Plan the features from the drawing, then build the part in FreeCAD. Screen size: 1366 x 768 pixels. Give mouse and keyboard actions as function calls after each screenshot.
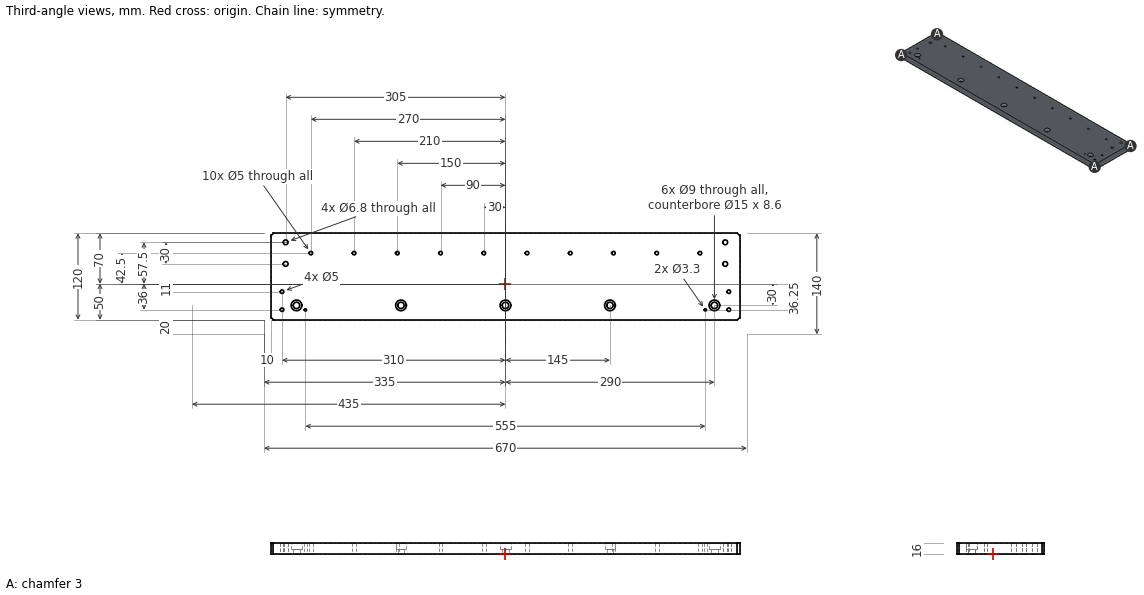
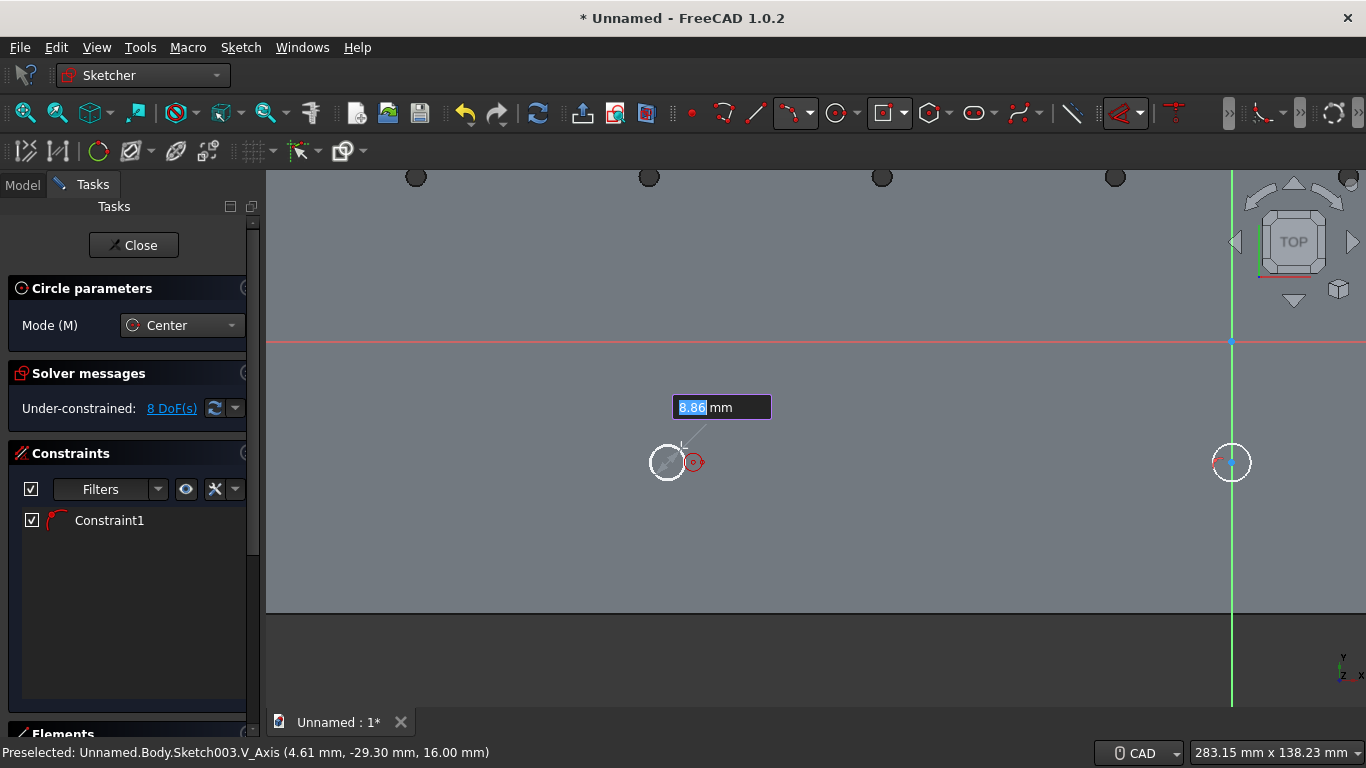
click(681, 446)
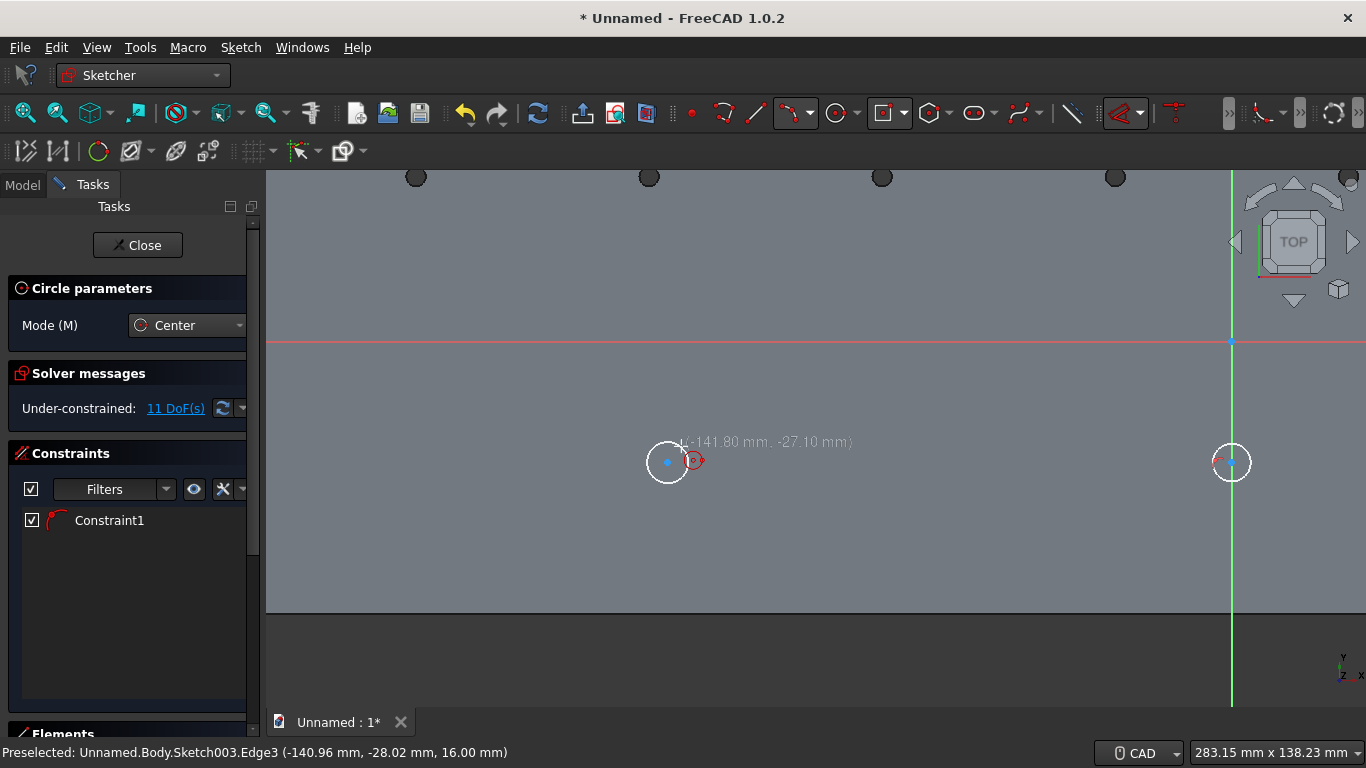
scroll(681, 448, down, 7)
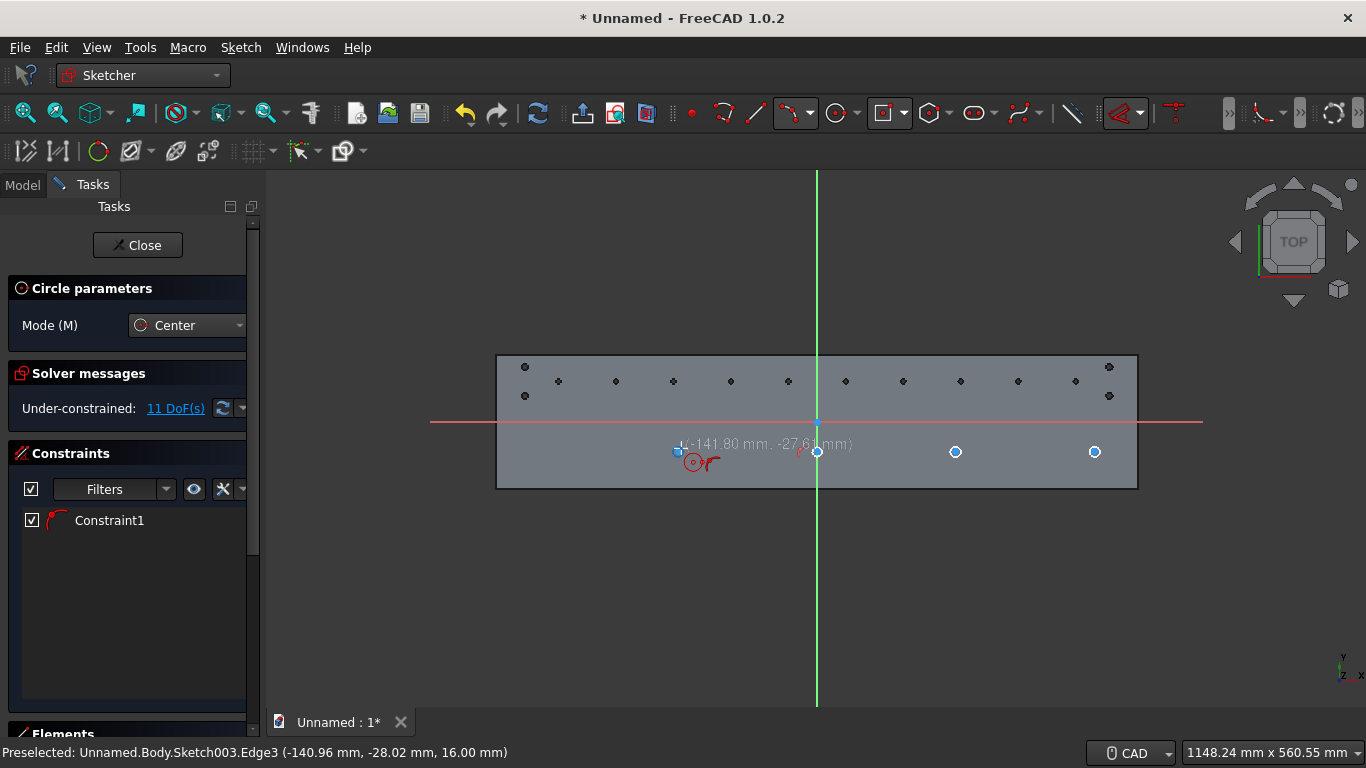
scroll(539, 451, up, 9)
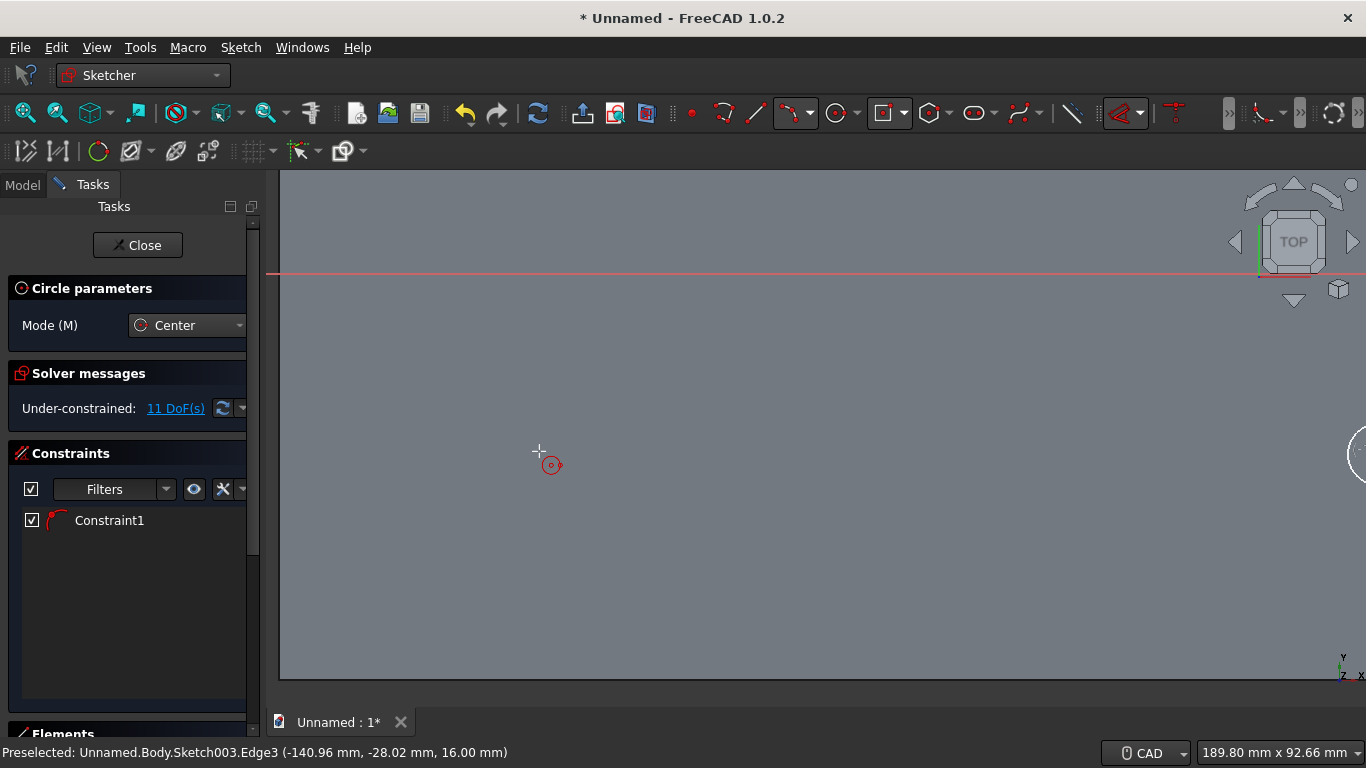
scroll(539, 451, down, 9)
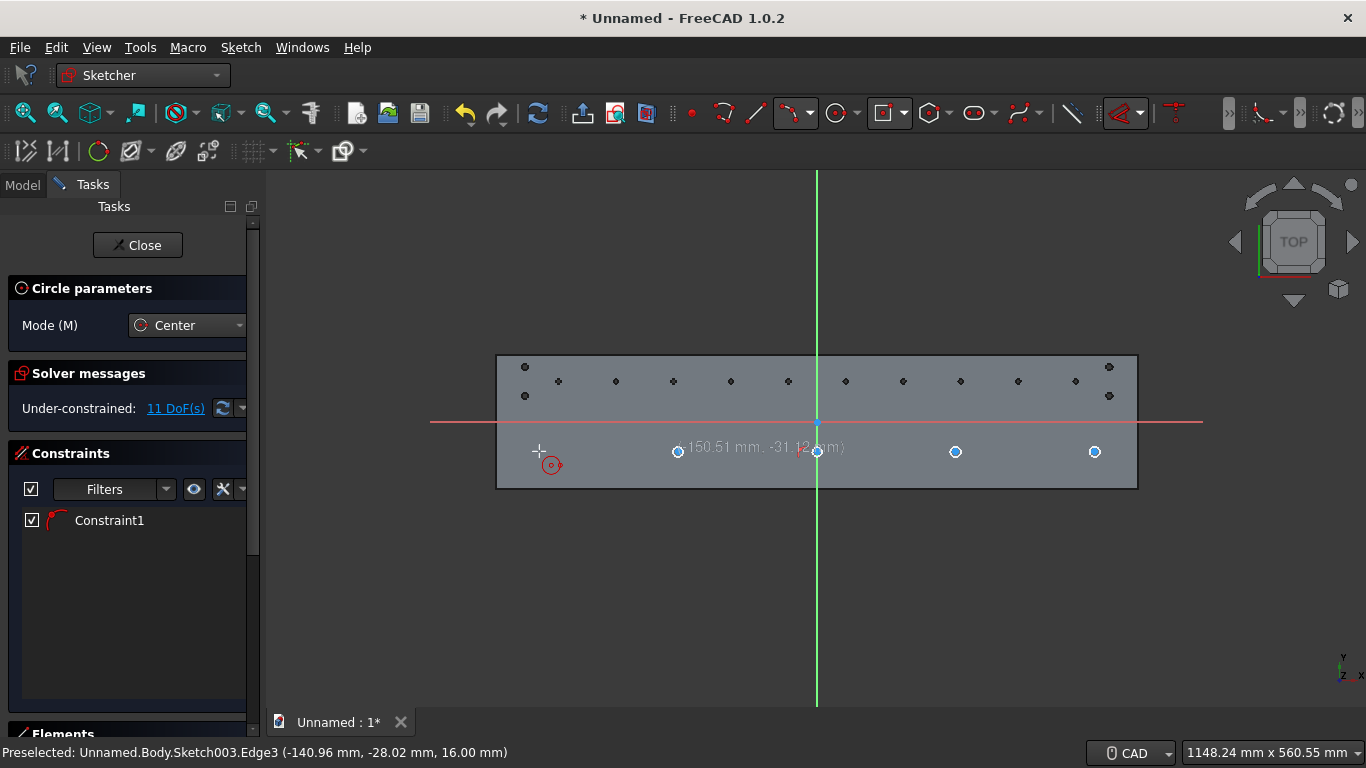
click(539, 451)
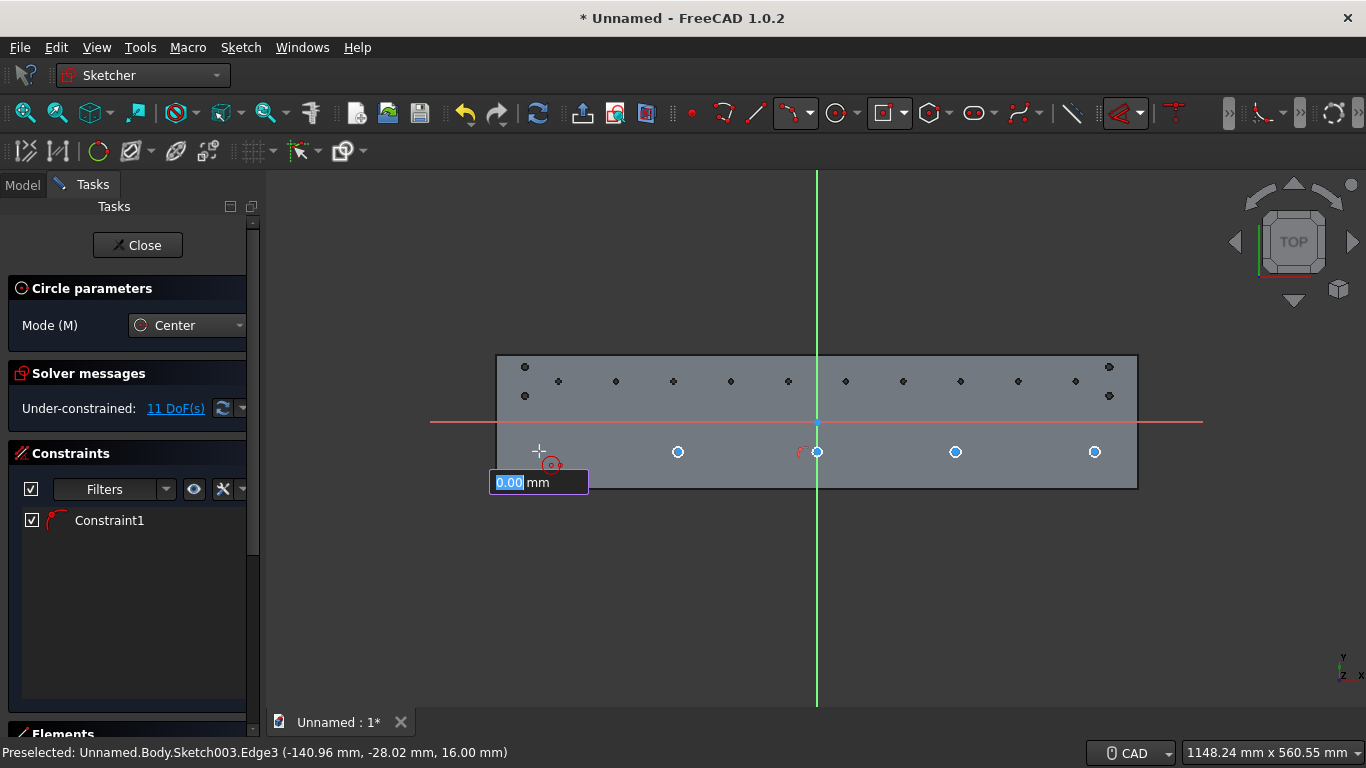
scroll(542, 448, up, 7)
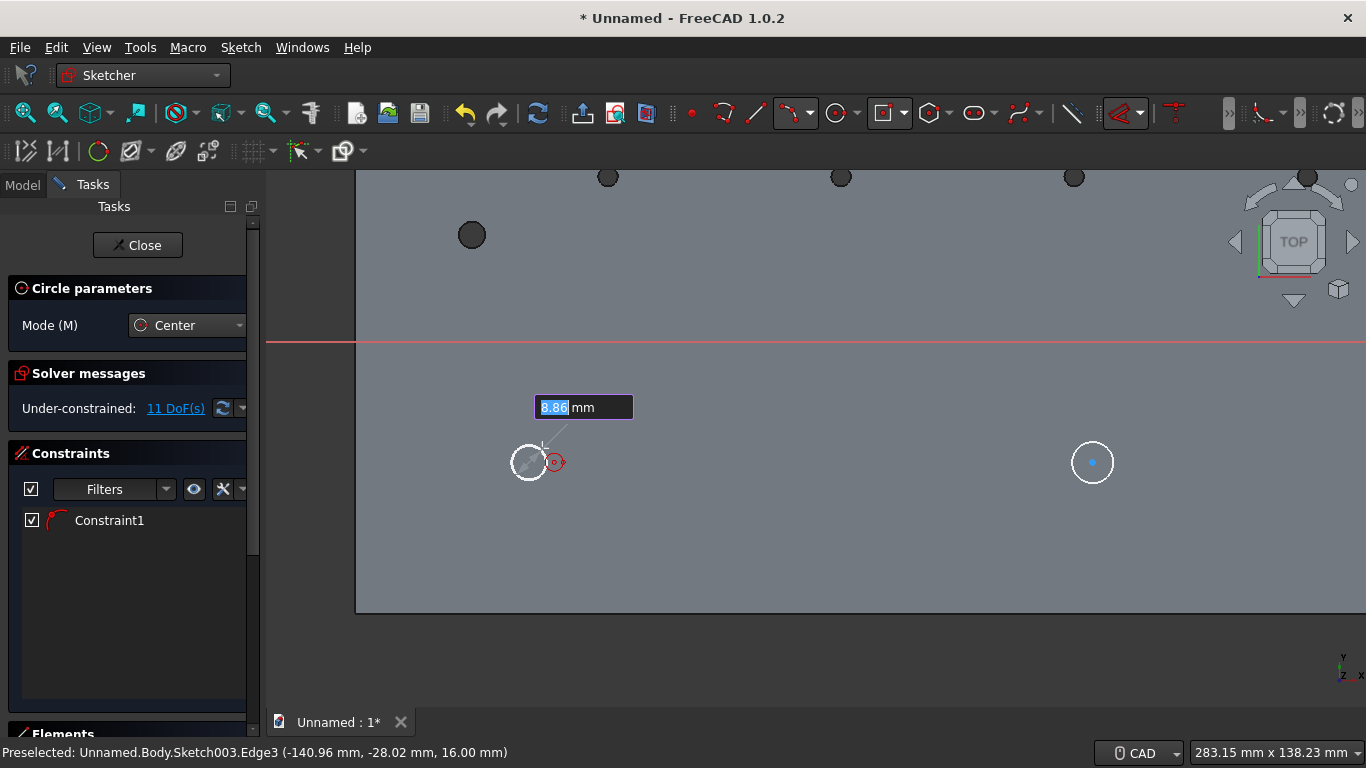
click(543, 446)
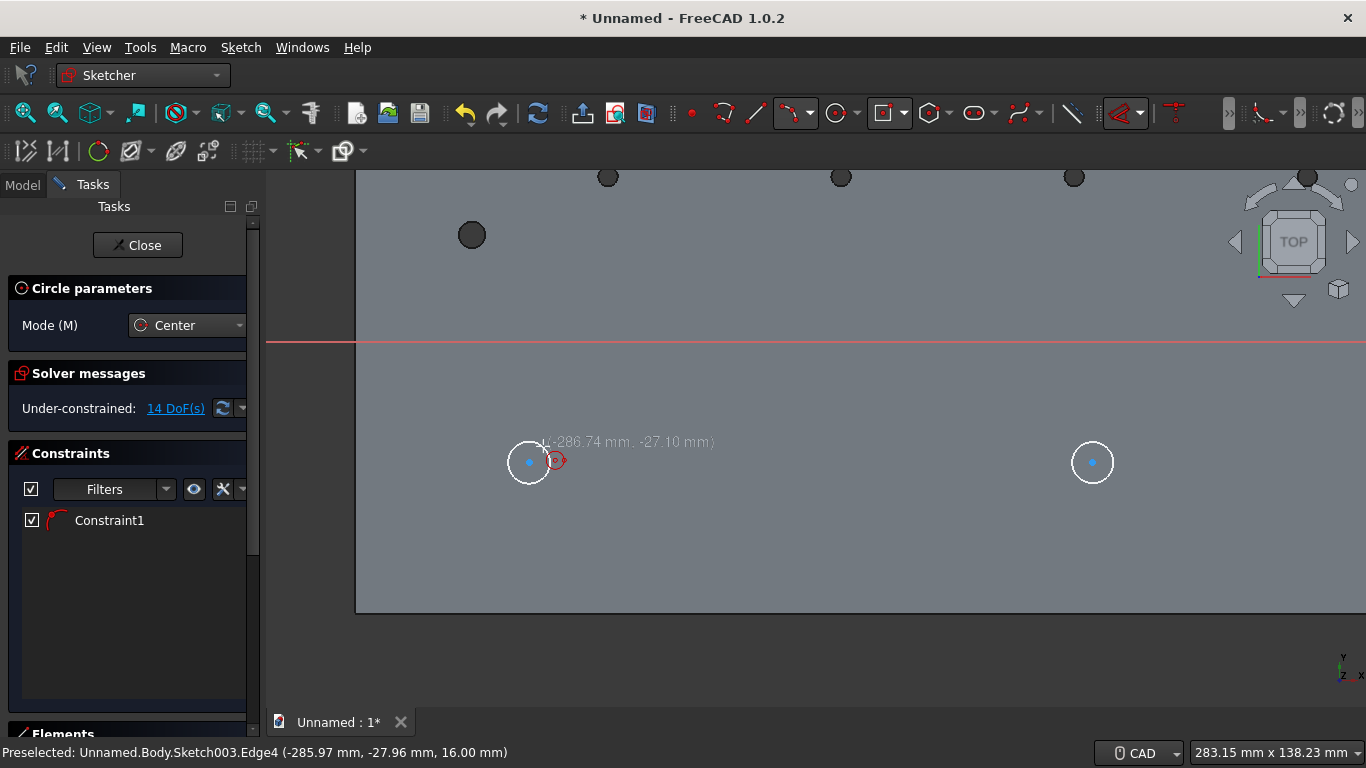
scroll(542, 448, down, 7)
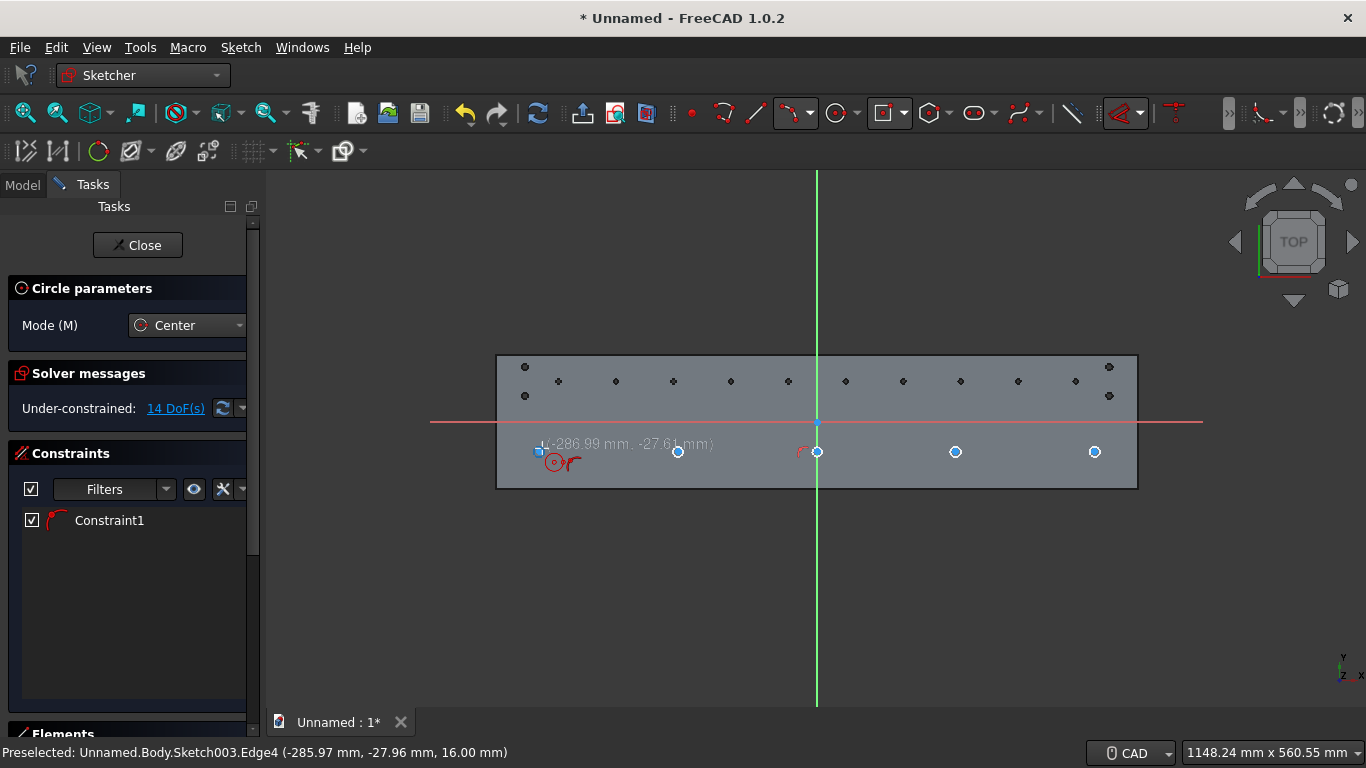
scroll(400, 451, up, 9)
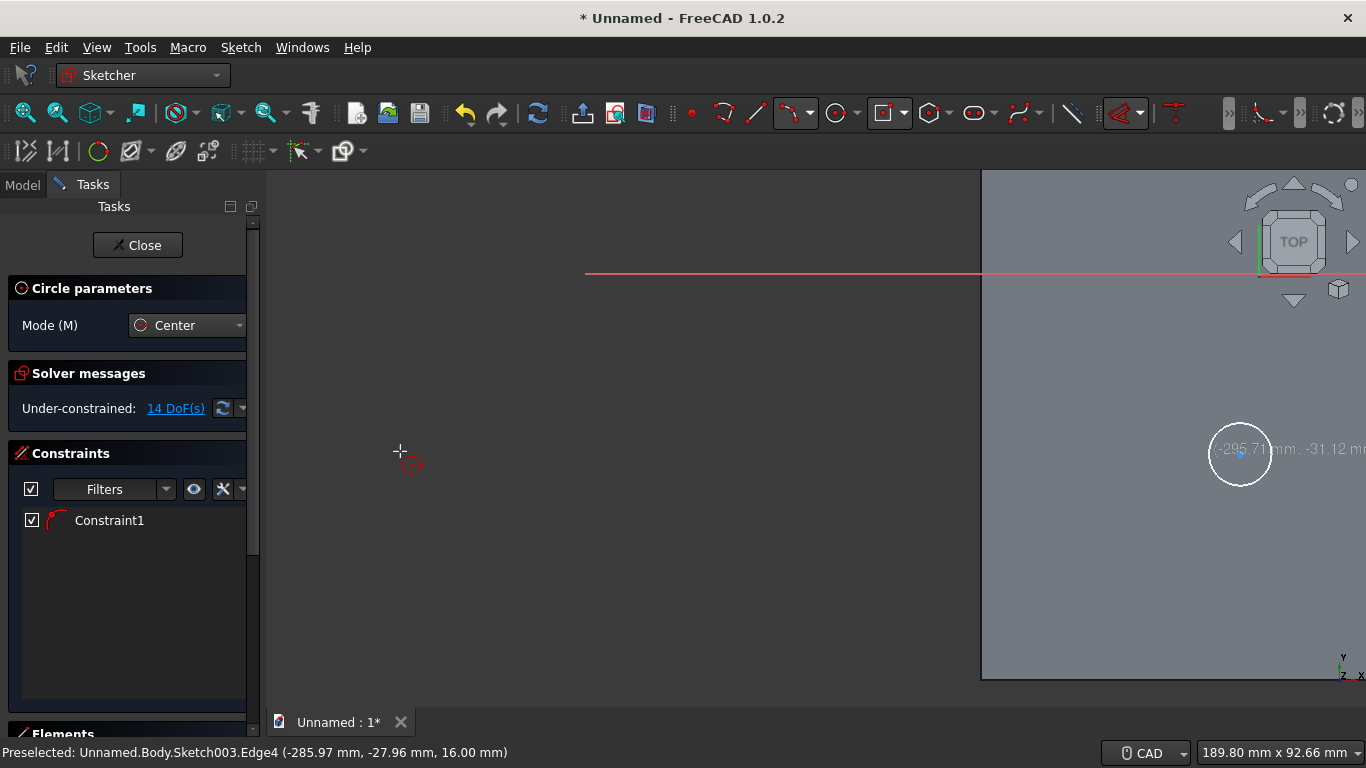
scroll(400, 451, down, 9)